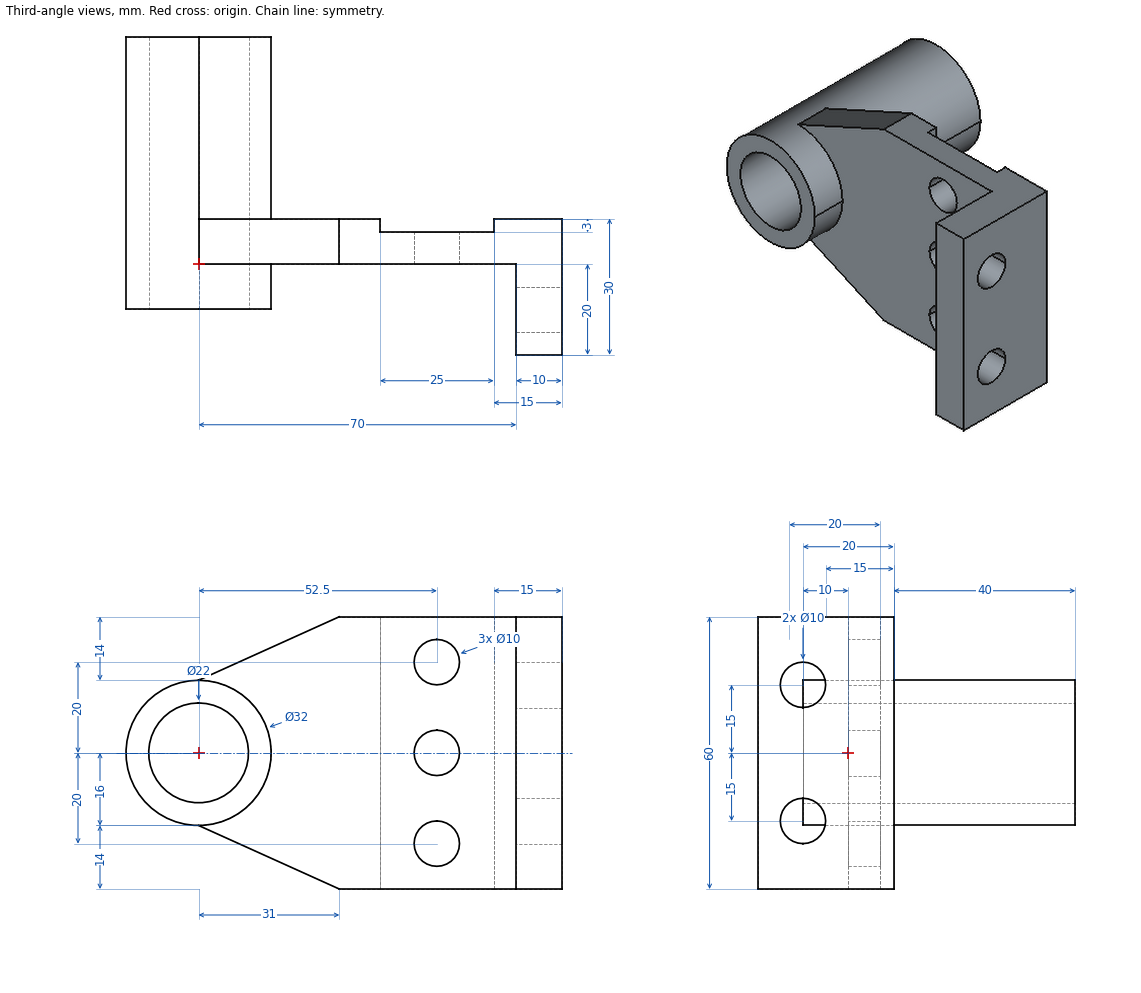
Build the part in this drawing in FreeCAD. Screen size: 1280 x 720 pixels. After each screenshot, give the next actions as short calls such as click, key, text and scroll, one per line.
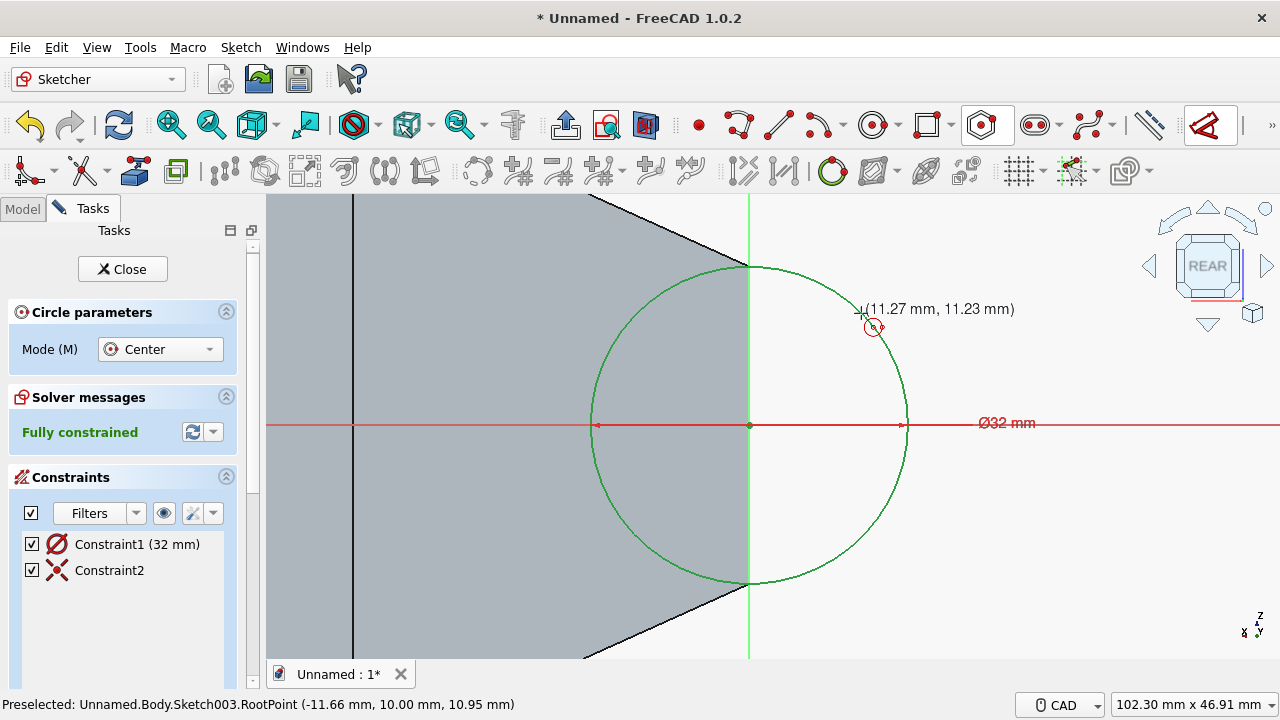
click(749, 425)
move(826, 348)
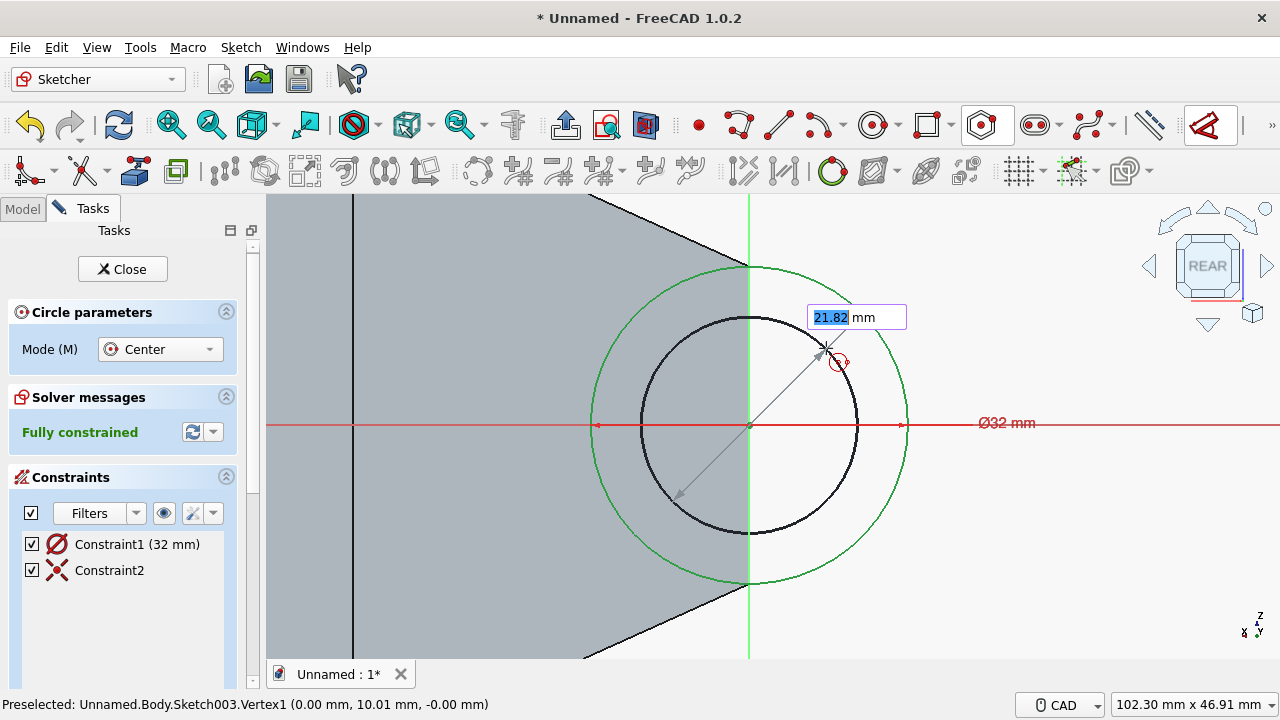
text(22)
key(Return)
key(Escape)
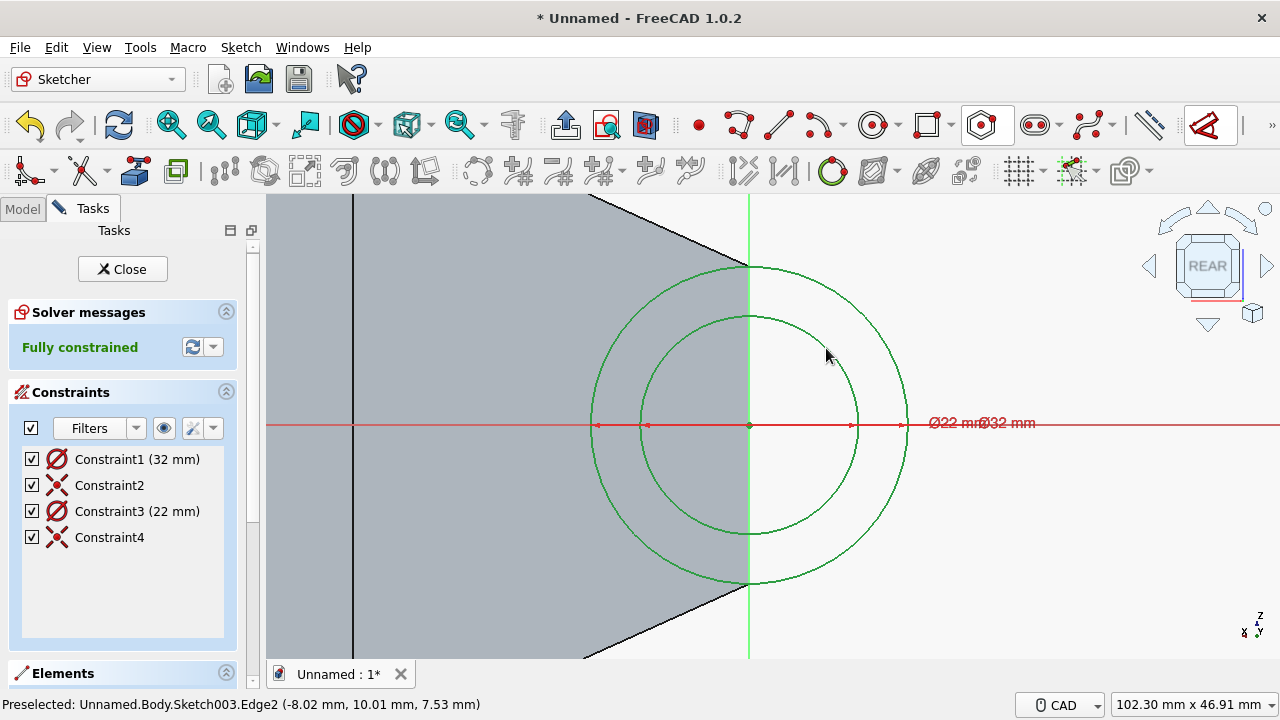
click(123, 269)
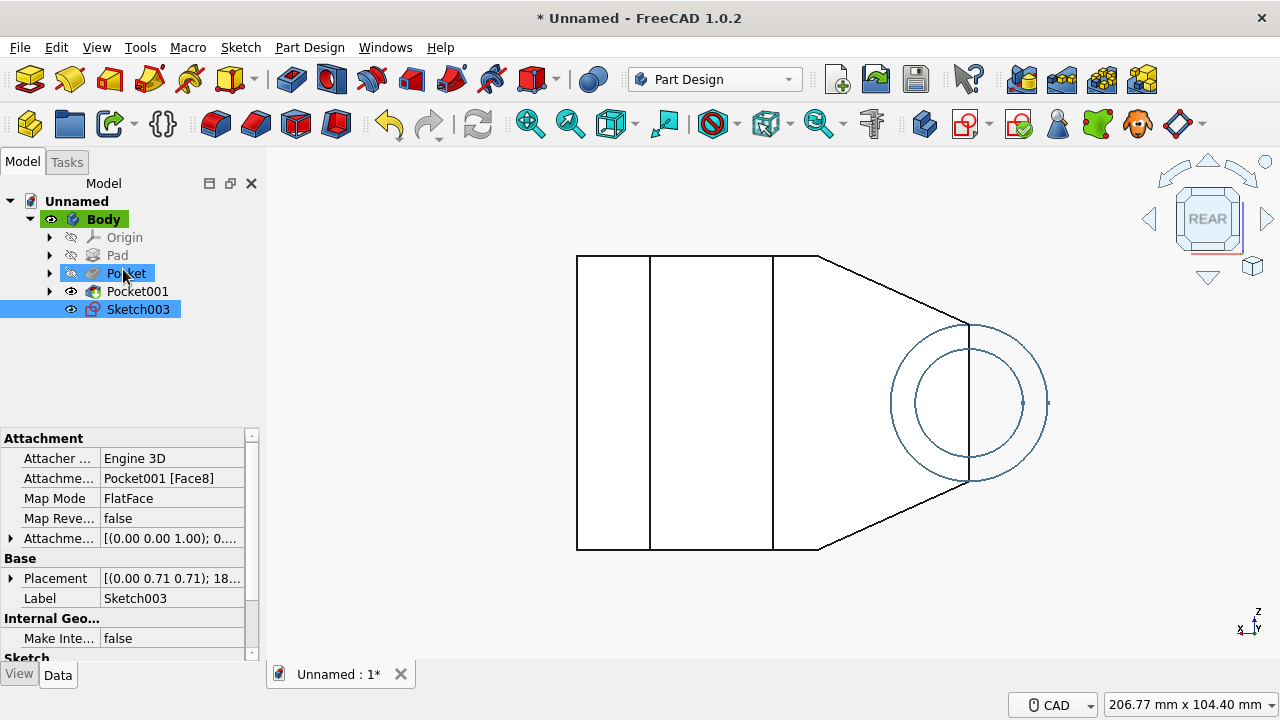
click(30, 80)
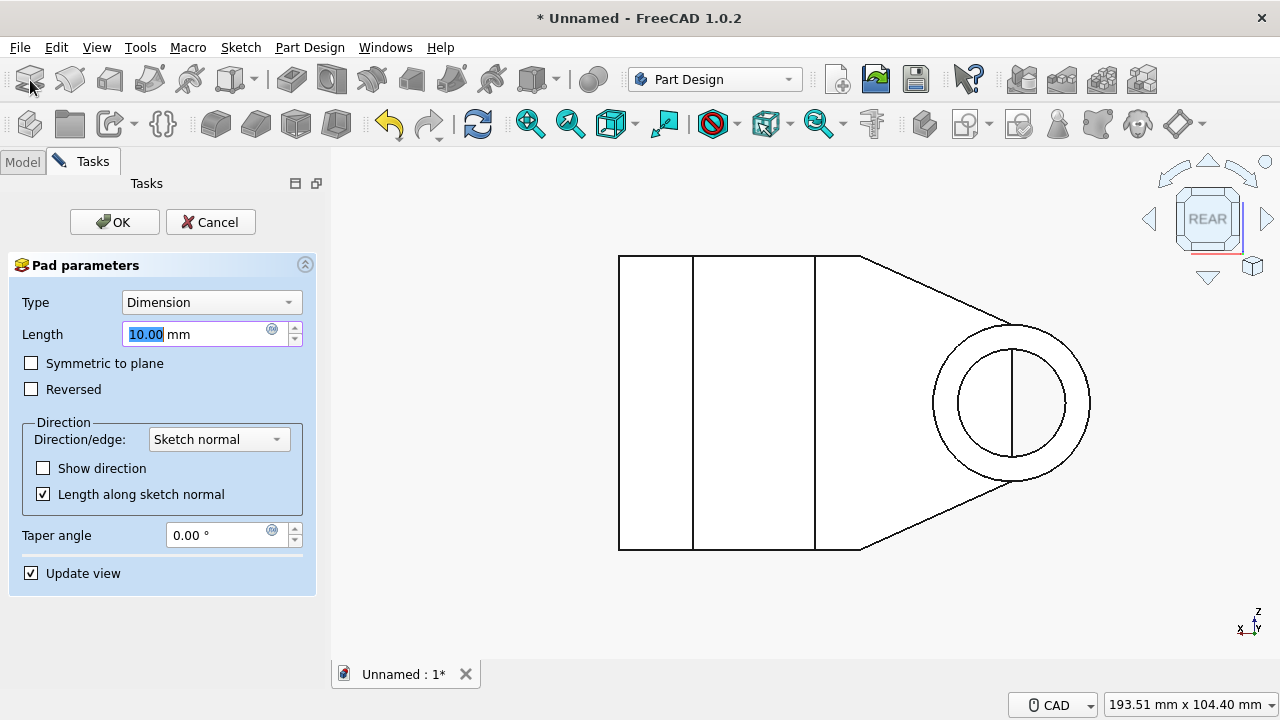
text(40)
key(Tab)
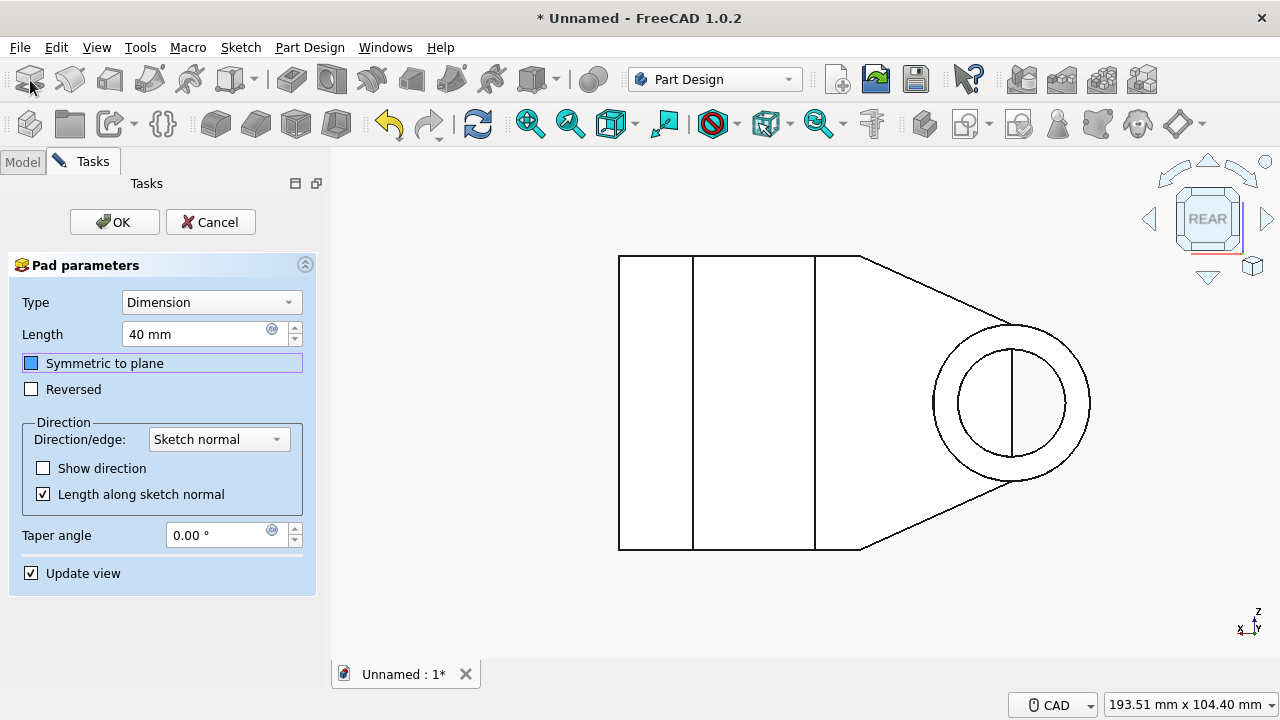
click(115, 222)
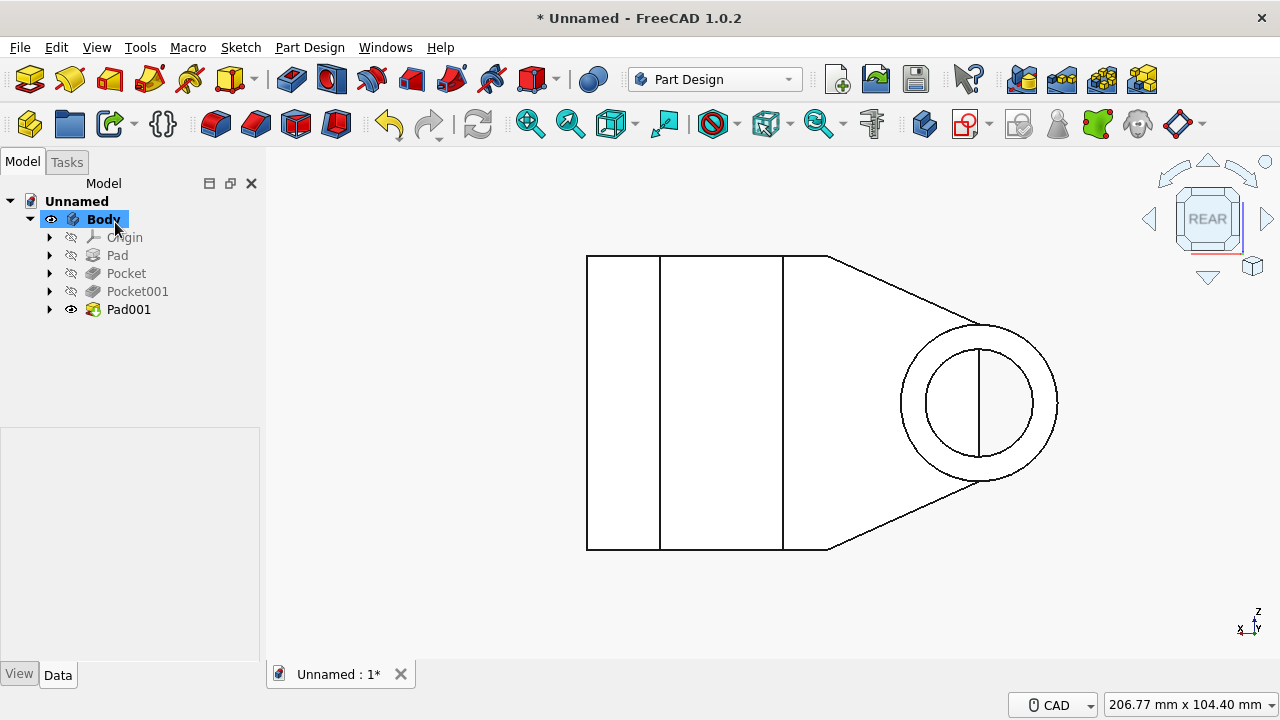
click(50, 237)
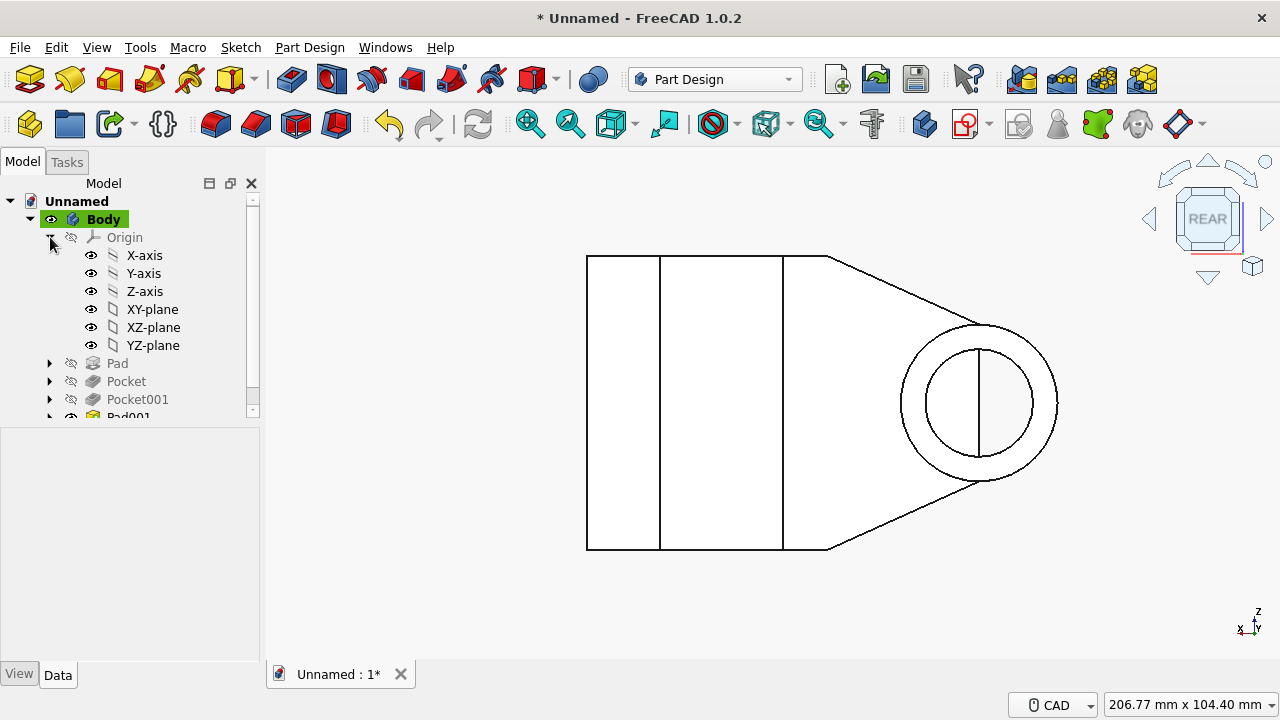
click(136, 327)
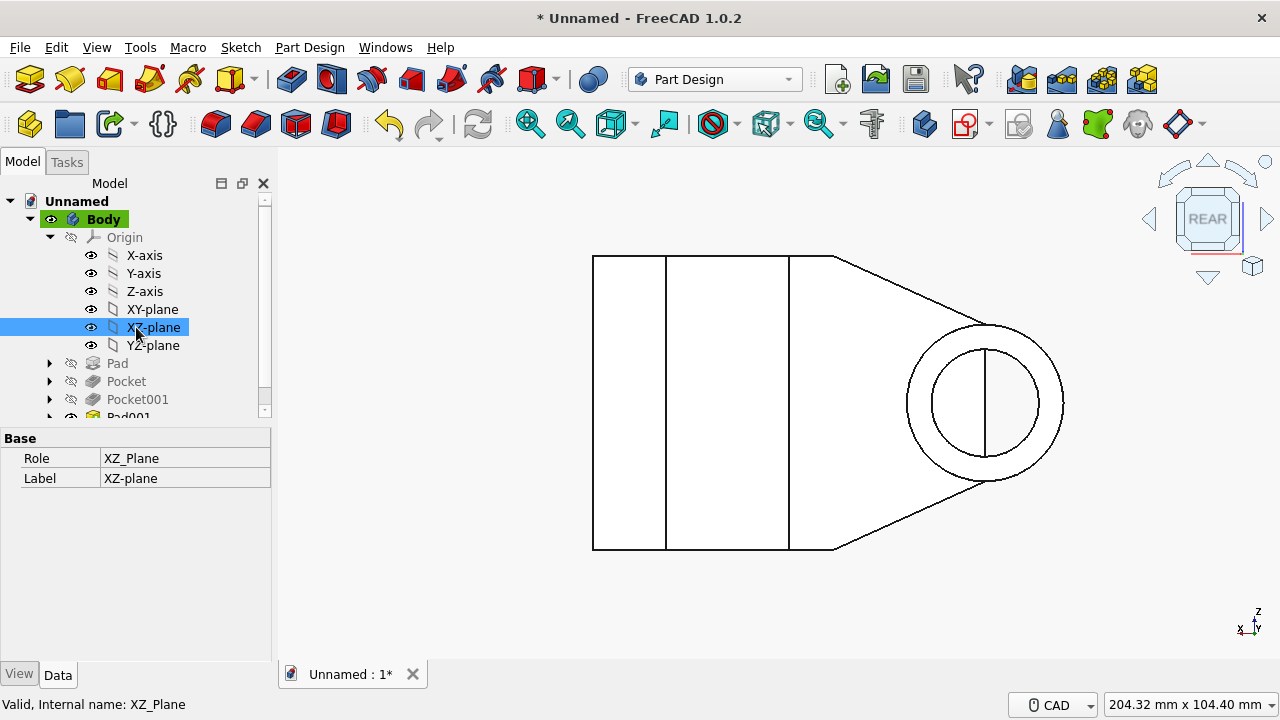
click(1178, 124)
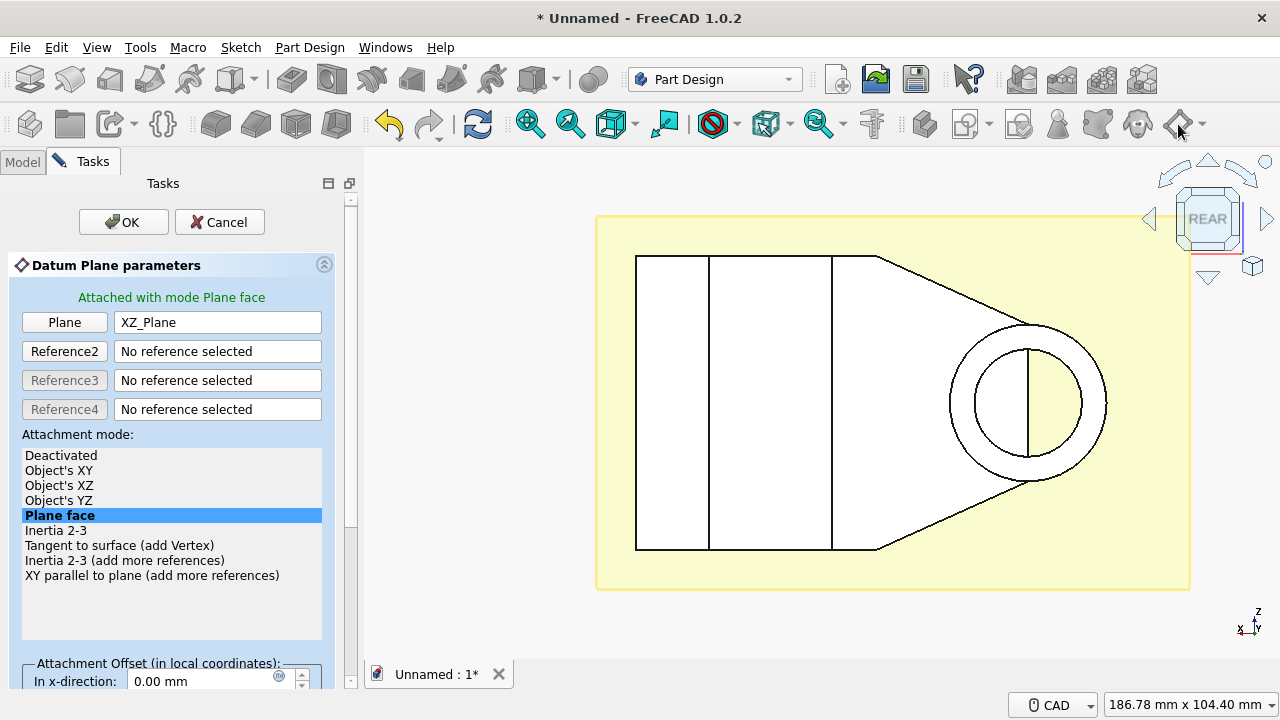
scroll(351, 440, down, 3)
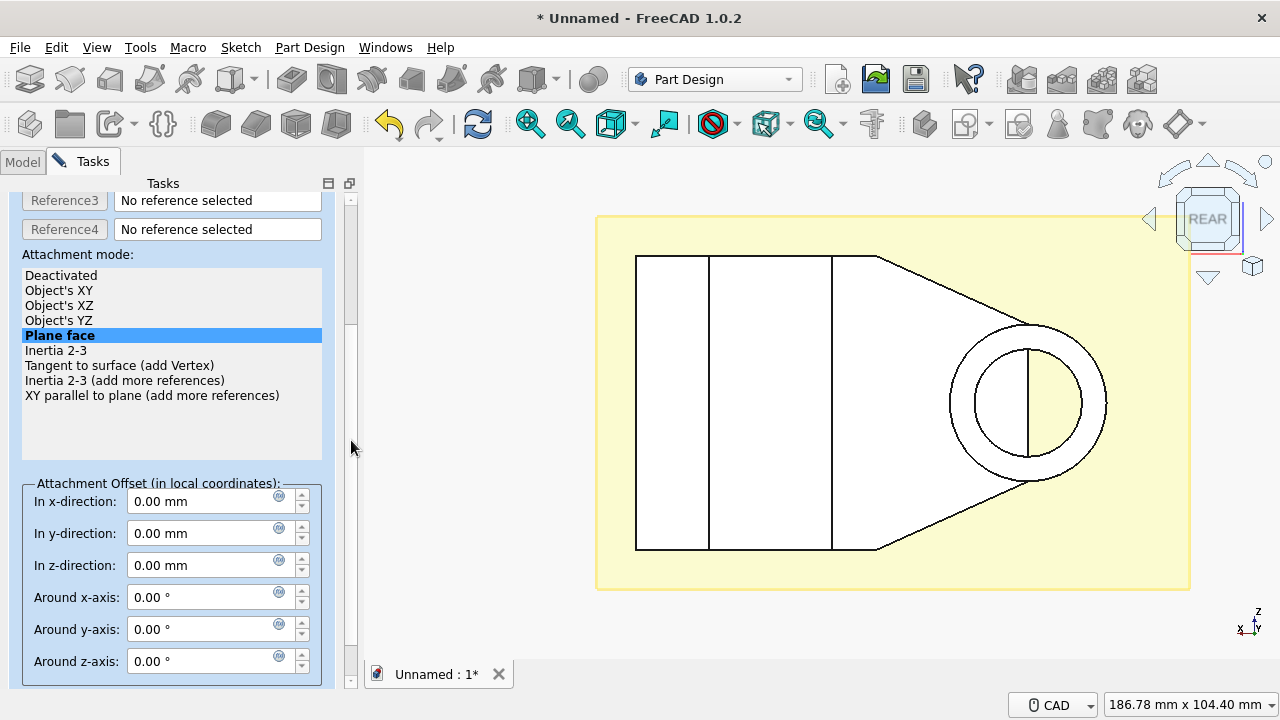
triple_click(210, 565)